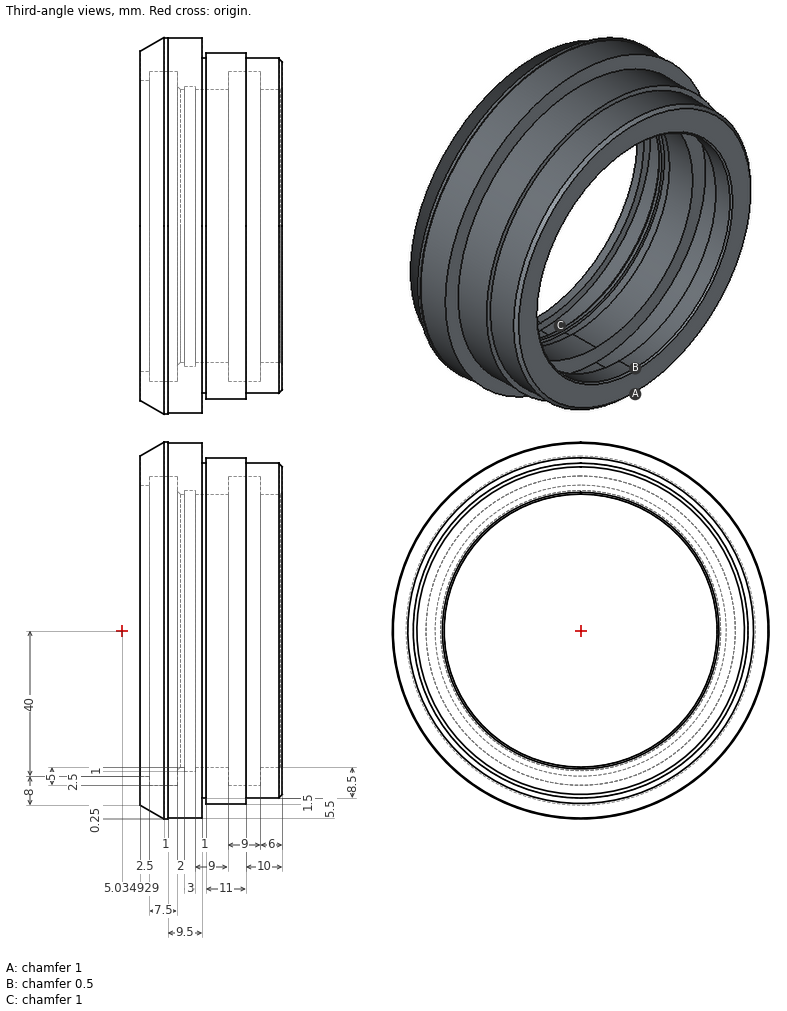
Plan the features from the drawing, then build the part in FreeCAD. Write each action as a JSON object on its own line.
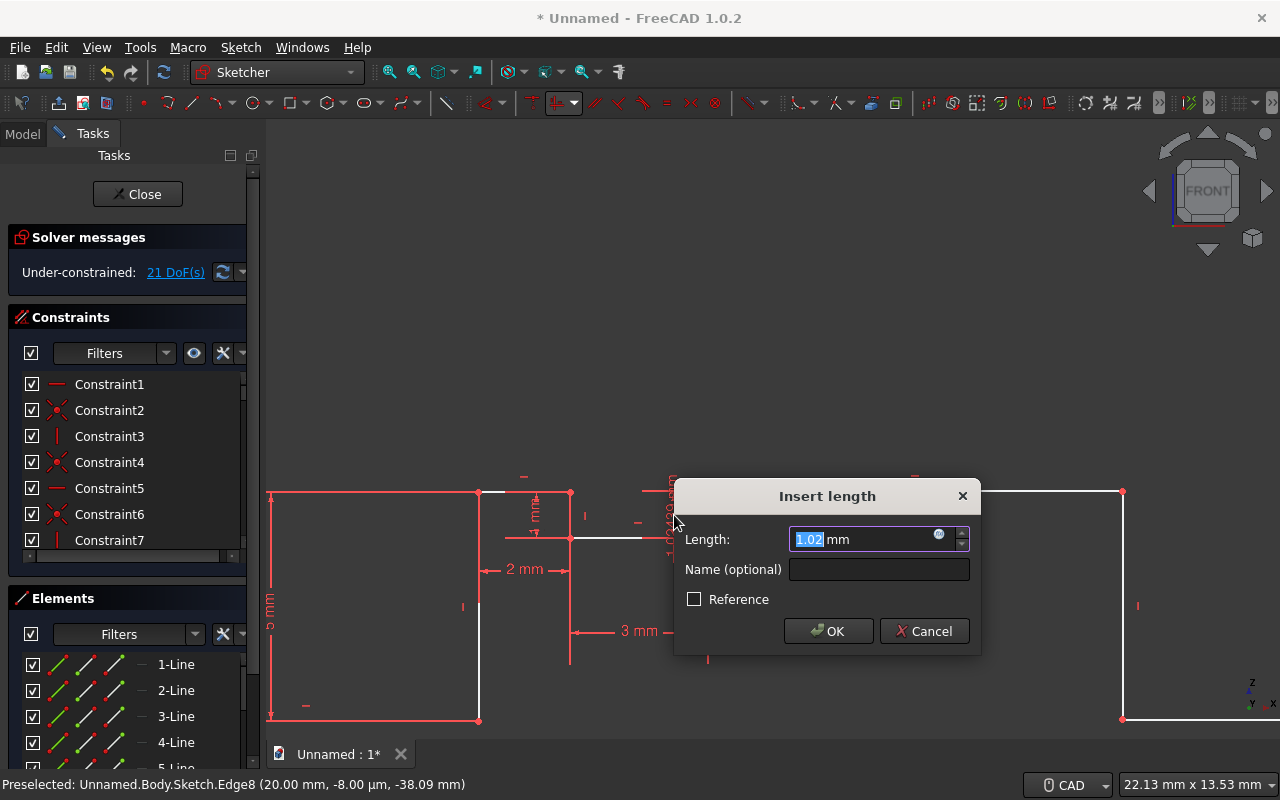
{"action": "type", "text": "1"}
{"action": "key", "text": "Return"}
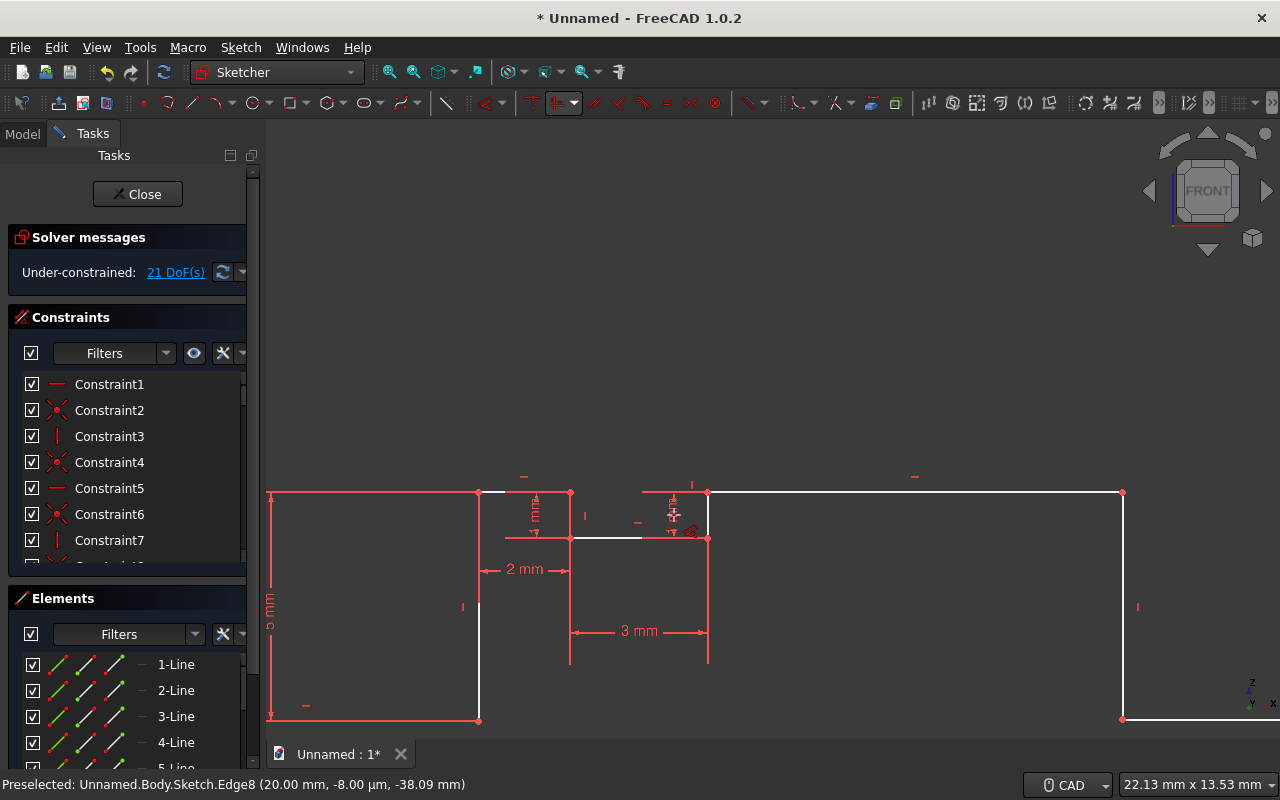
{"action": "scroll", "coordinate": [686, 523], "scroll_direction": "down", "scroll_amount": 9}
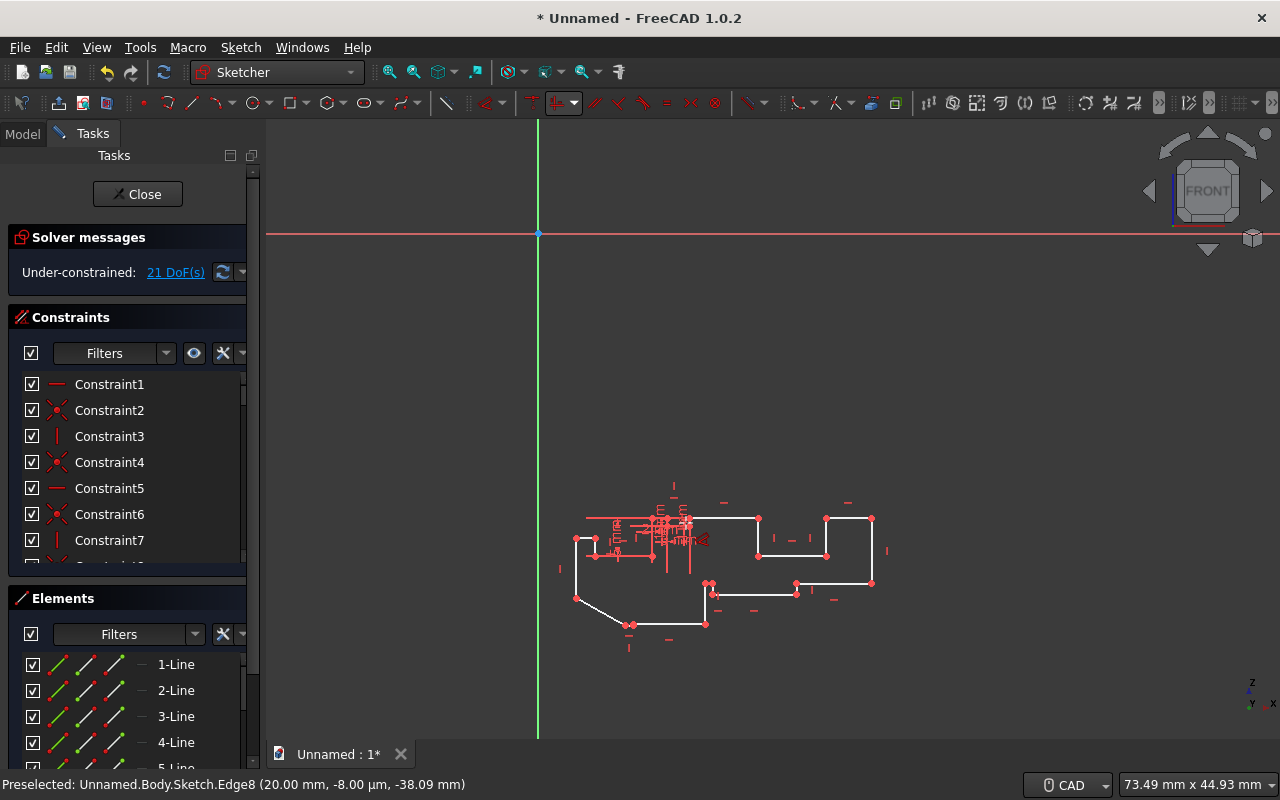
{"action": "left_click", "coordinate": [711, 518]}
{"action": "left_click", "coordinate": [724, 484]}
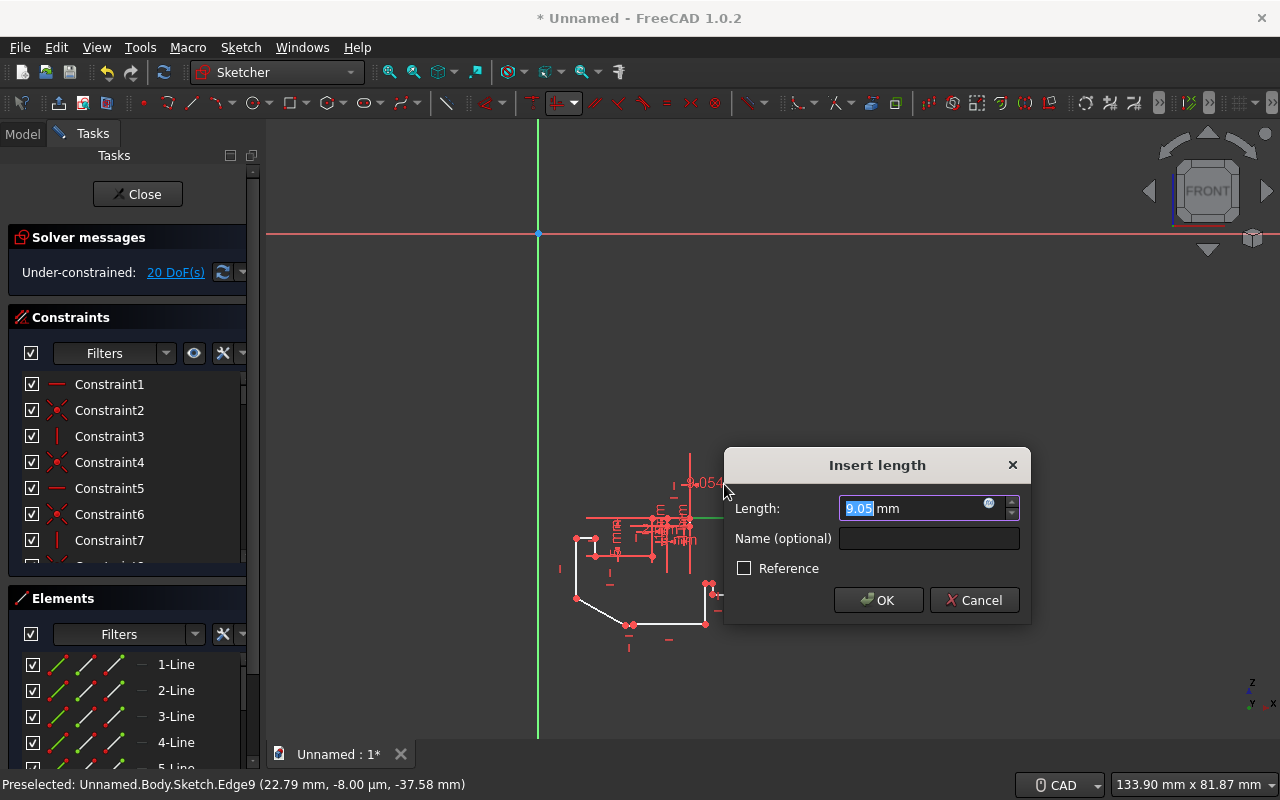
{"action": "type", "text": "9"}
{"action": "key", "text": "Return"}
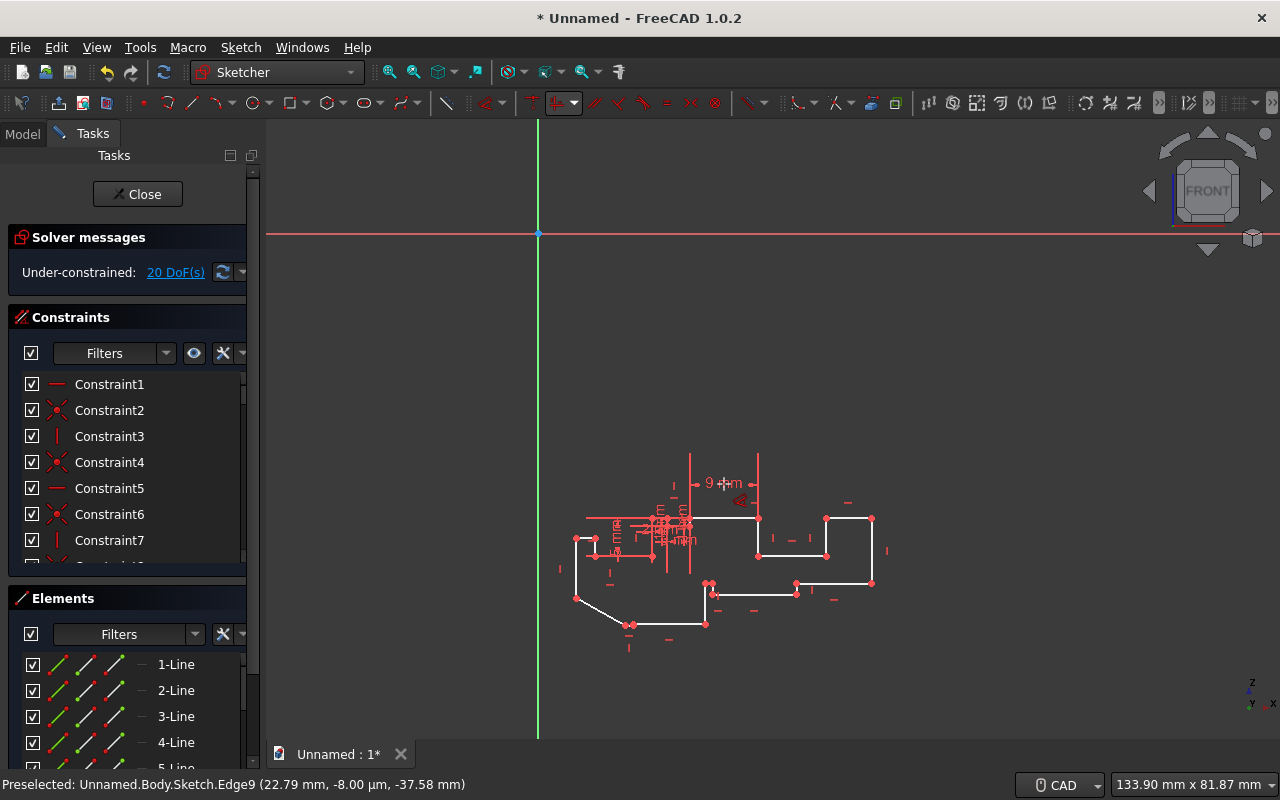
{"action": "scroll", "coordinate": [758, 530], "scroll_direction": "up", "scroll_amount": 2}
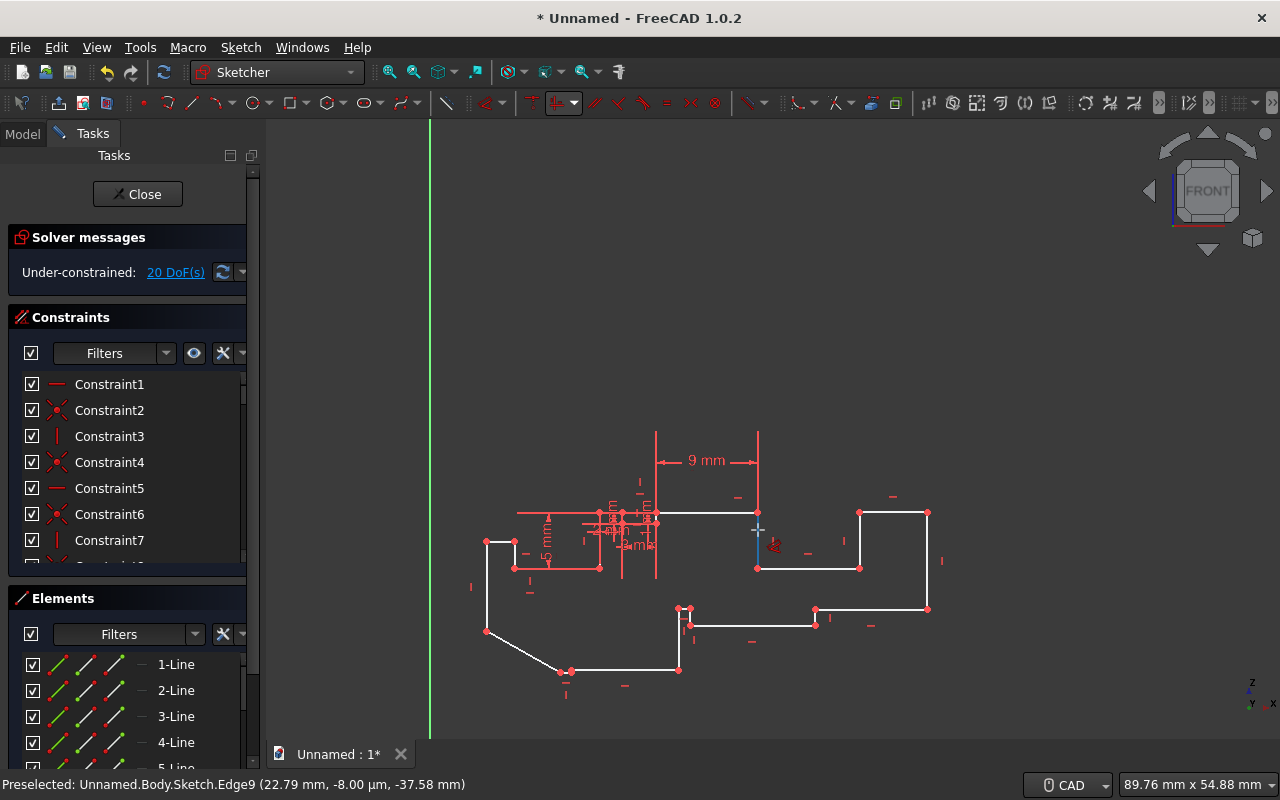
{"action": "left_click", "coordinate": [758, 529]}
{"action": "left_click", "coordinate": [792, 541]}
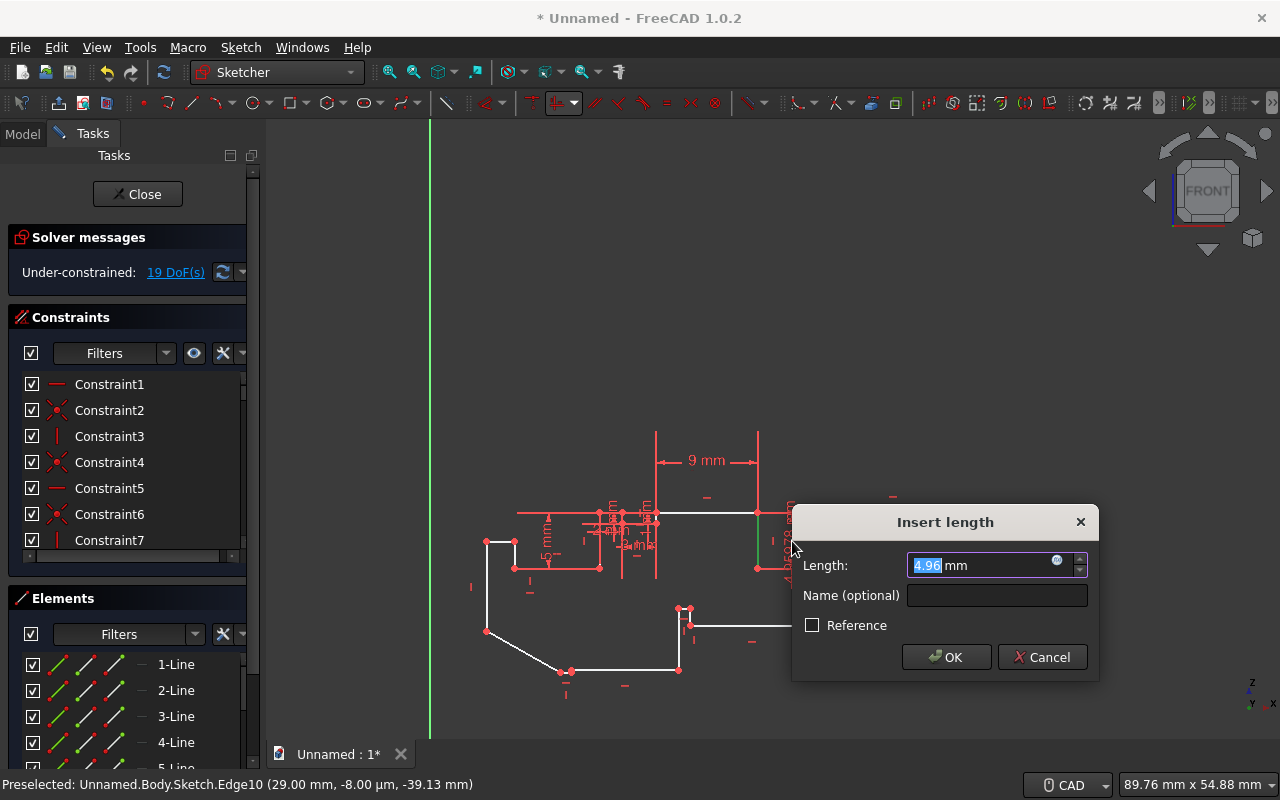
{"action": "type", "text": "5"}
{"action": "key", "text": "Return"}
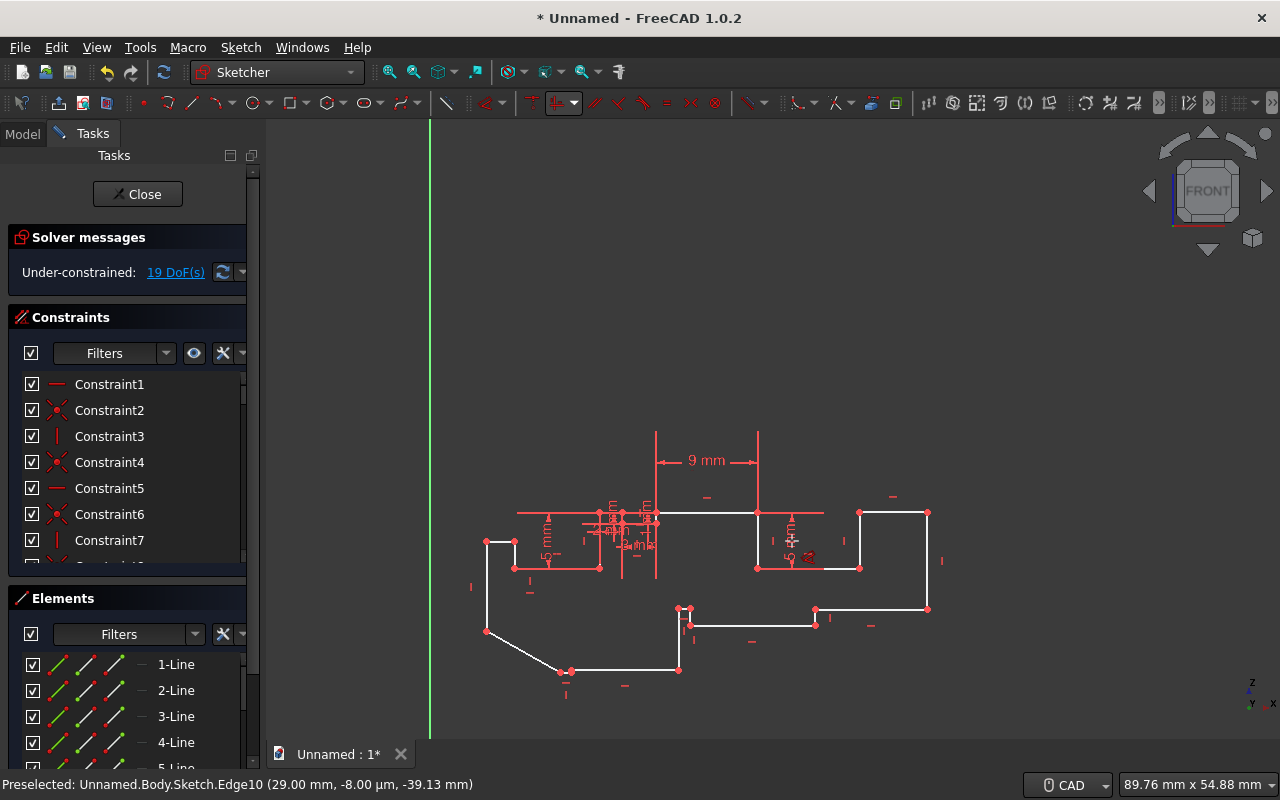
{"action": "left_click", "coordinate": [788, 569]}
{"action": "left_click", "coordinate": [785, 603]}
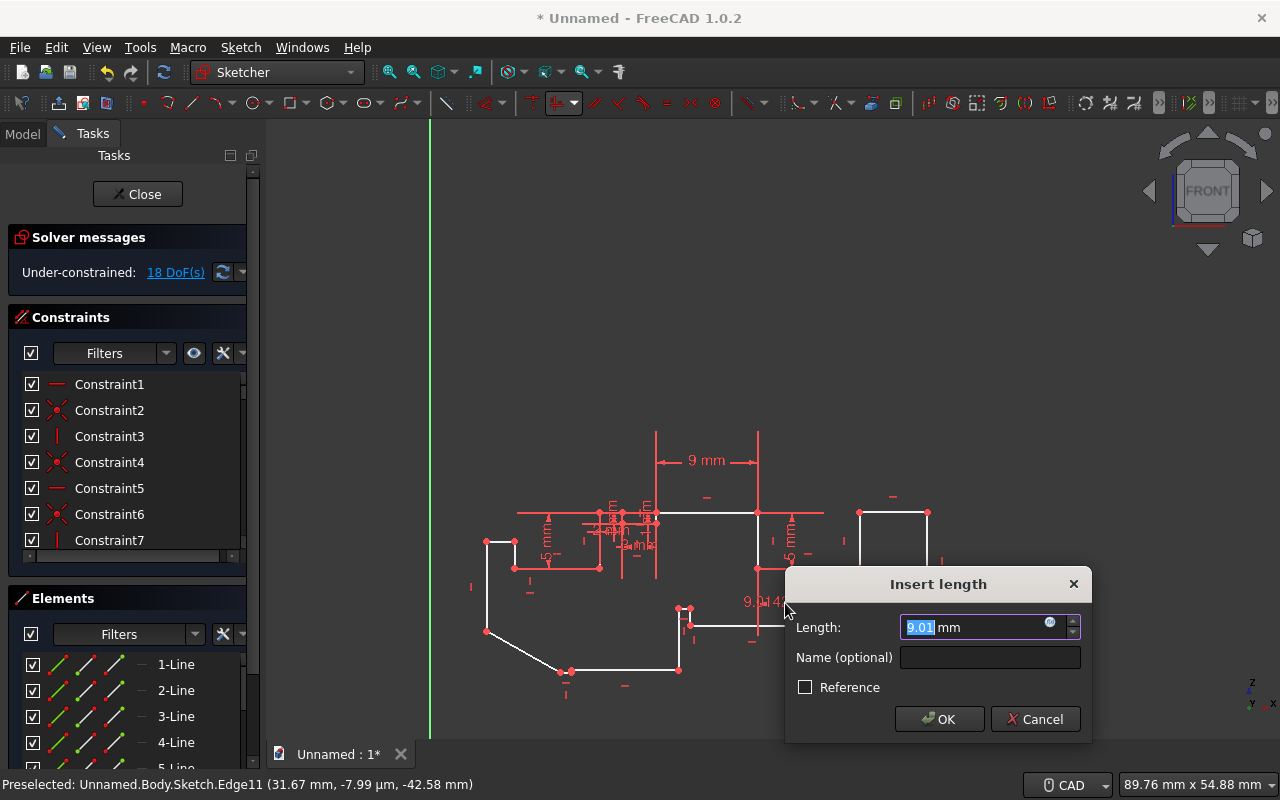
{"action": "type", "text": "9"}
{"action": "key", "text": "Return"}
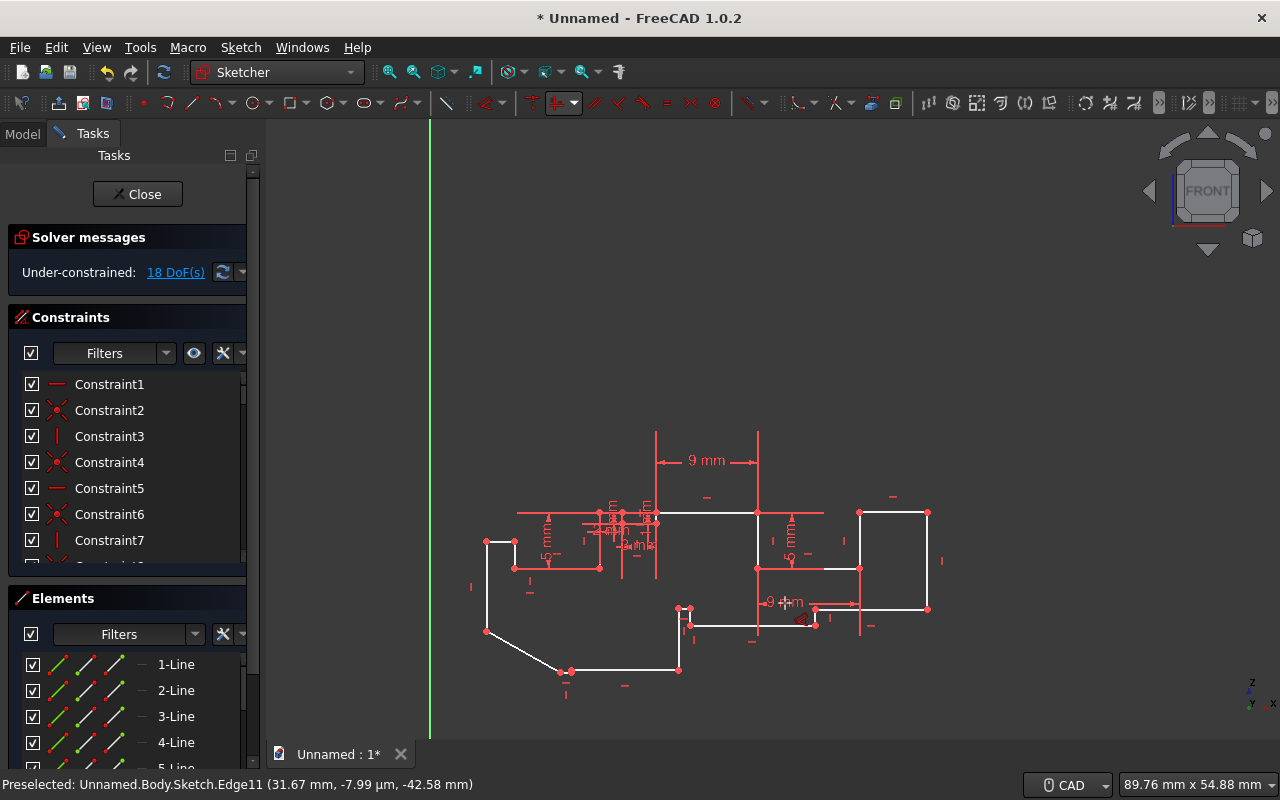
{"action": "left_click", "coordinate": [860, 552]}
{"action": "left_click", "coordinate": [894, 541]}